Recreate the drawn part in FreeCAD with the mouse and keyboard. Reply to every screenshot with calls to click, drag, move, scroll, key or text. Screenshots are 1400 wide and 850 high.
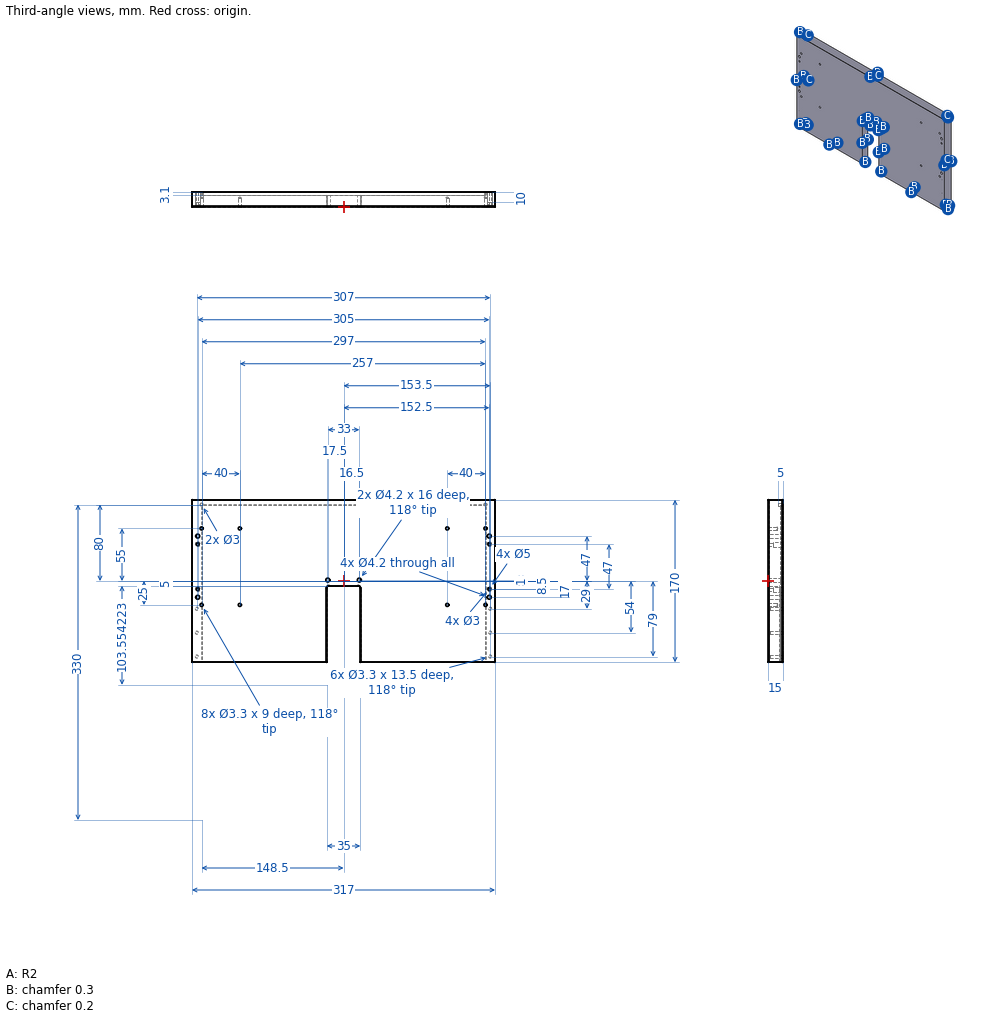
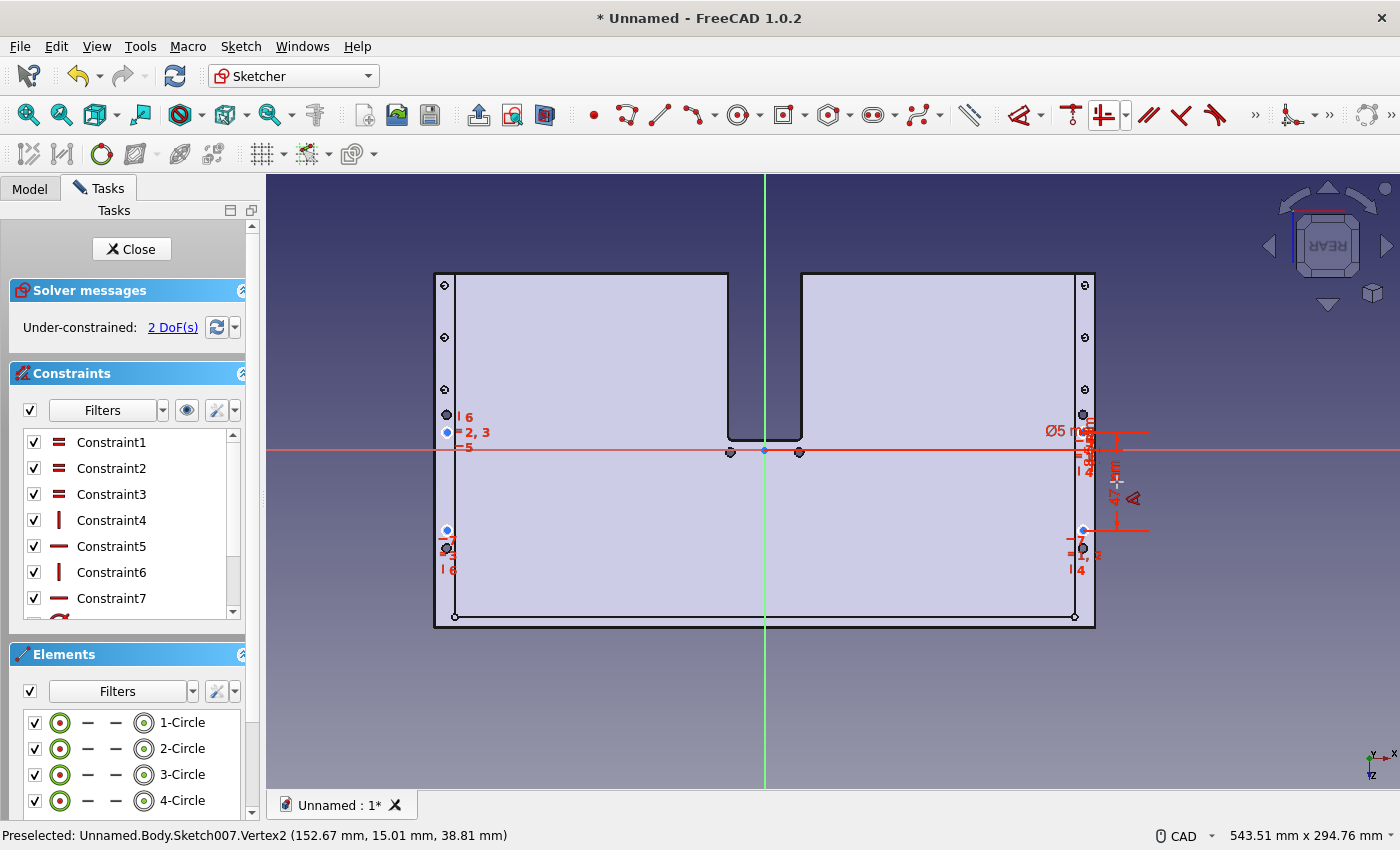
click(1083, 433)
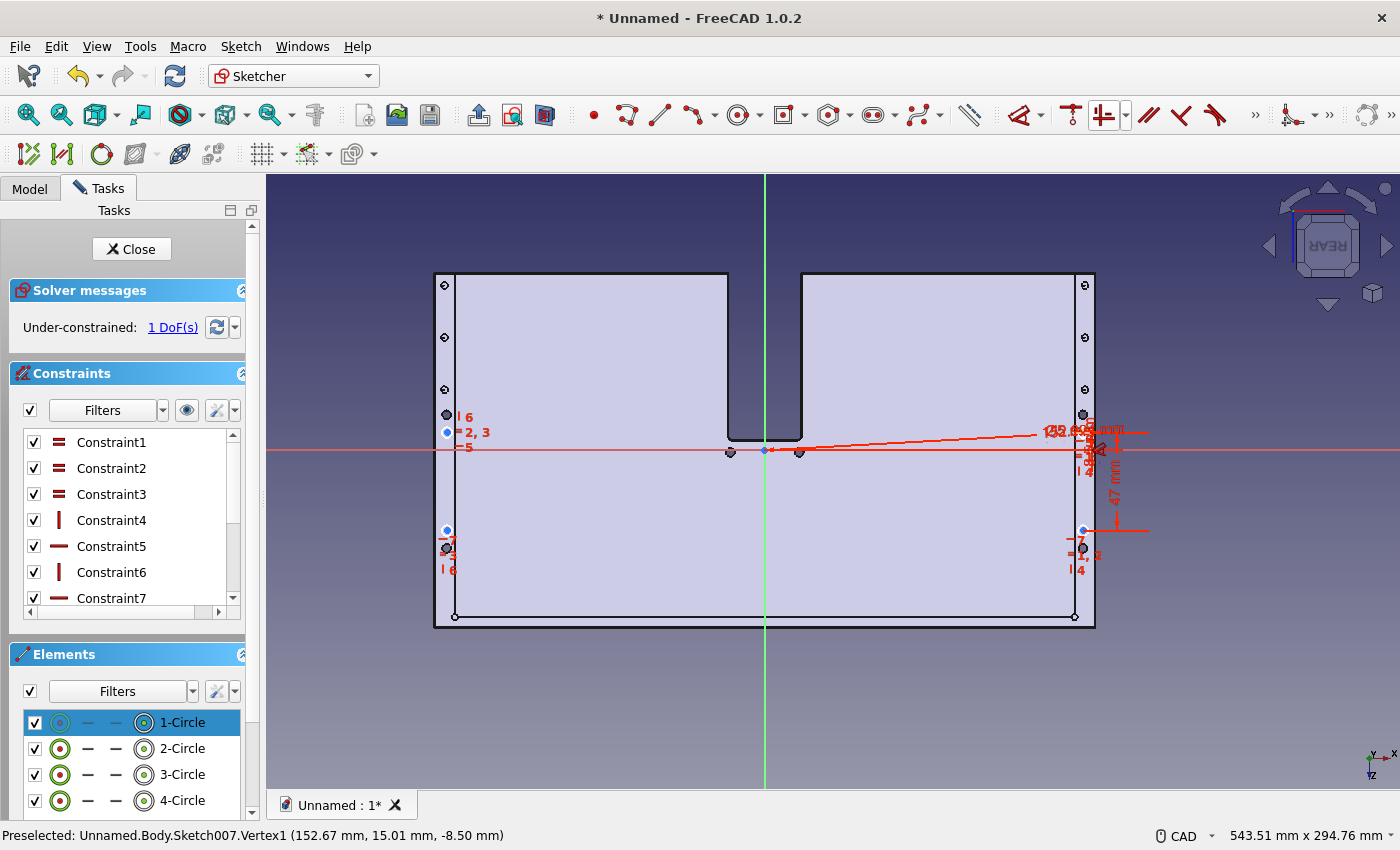
click(447, 433)
click(619, 399)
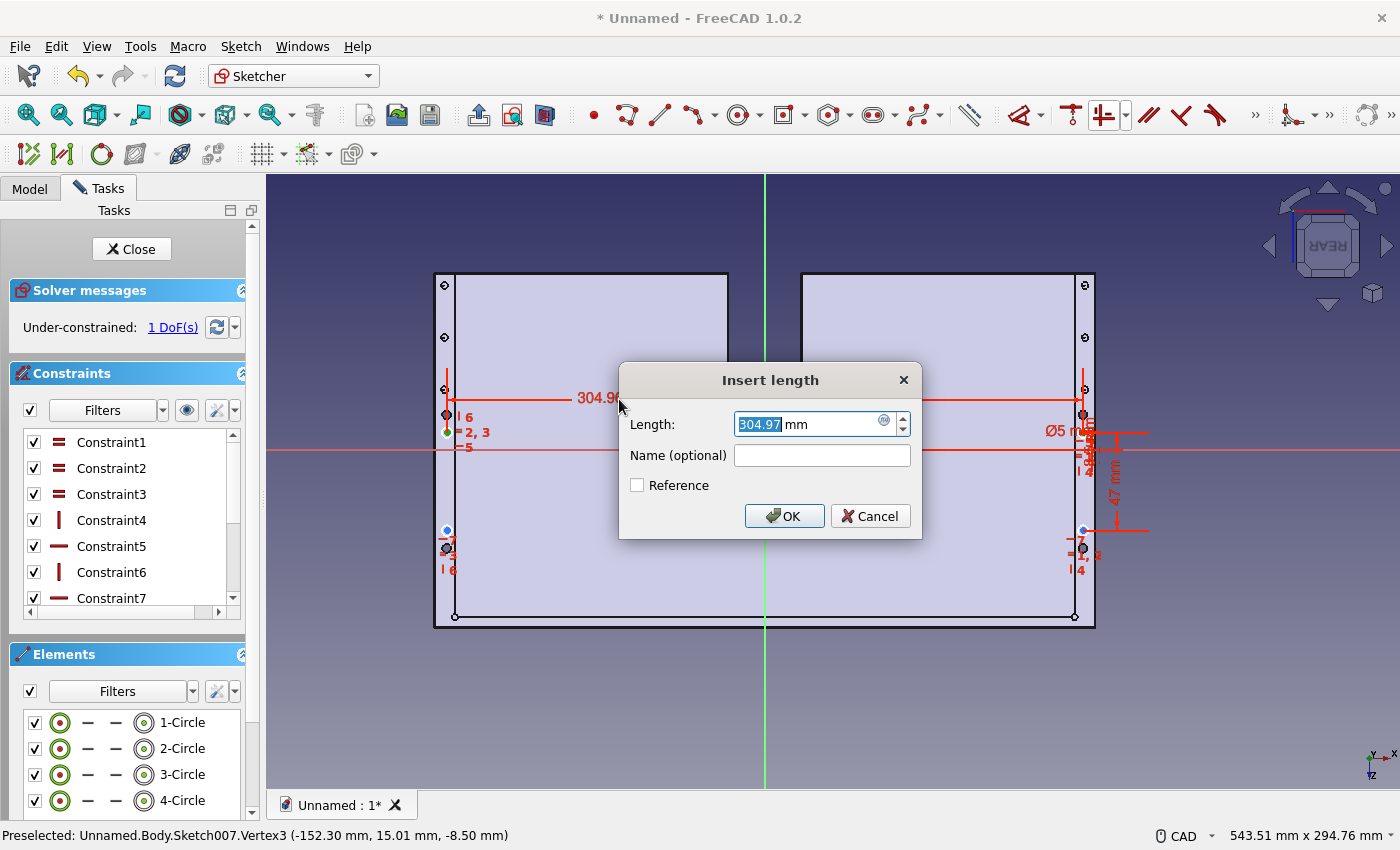
text(305)
key(Return)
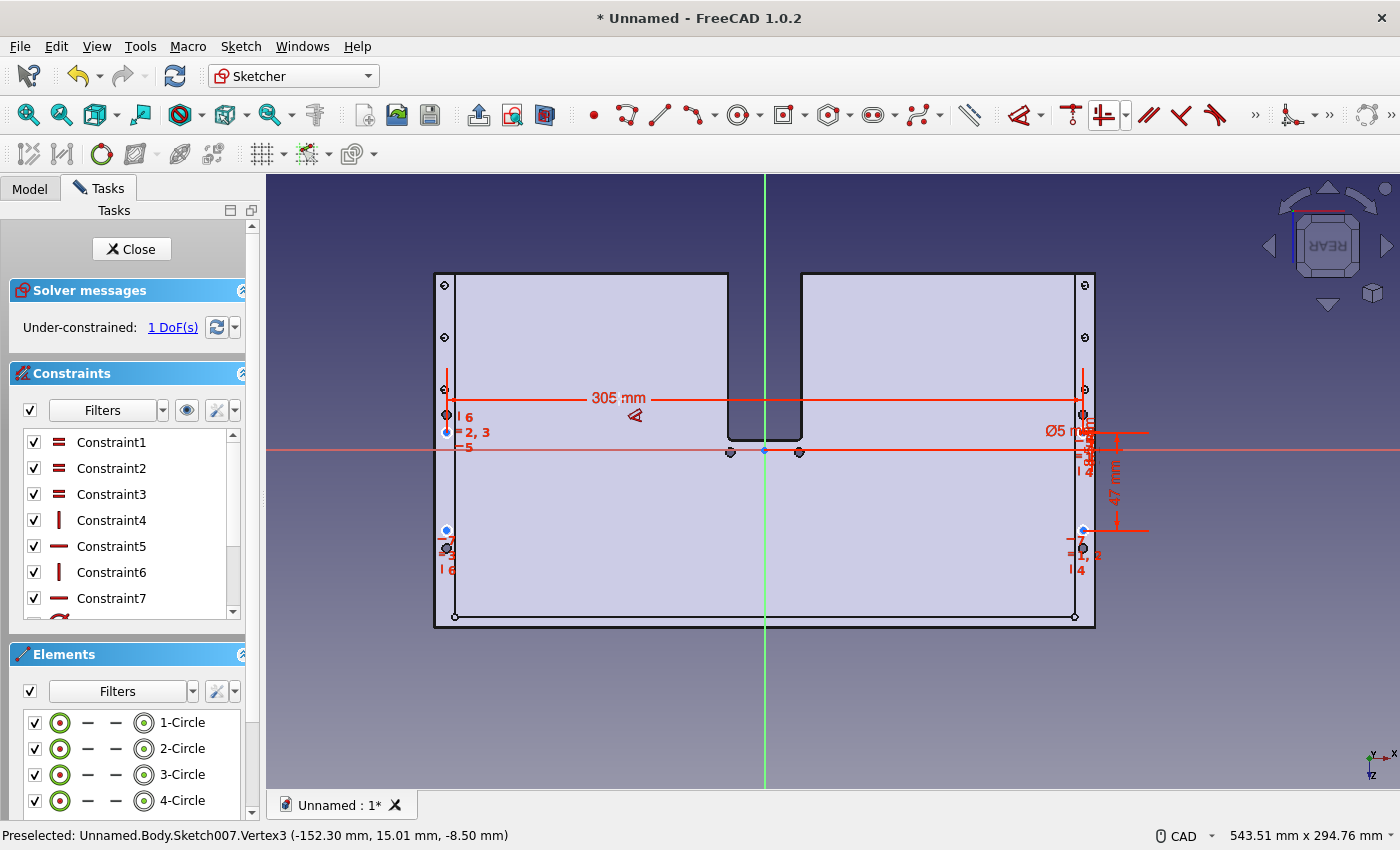
click(1083, 433)
click(924, 399)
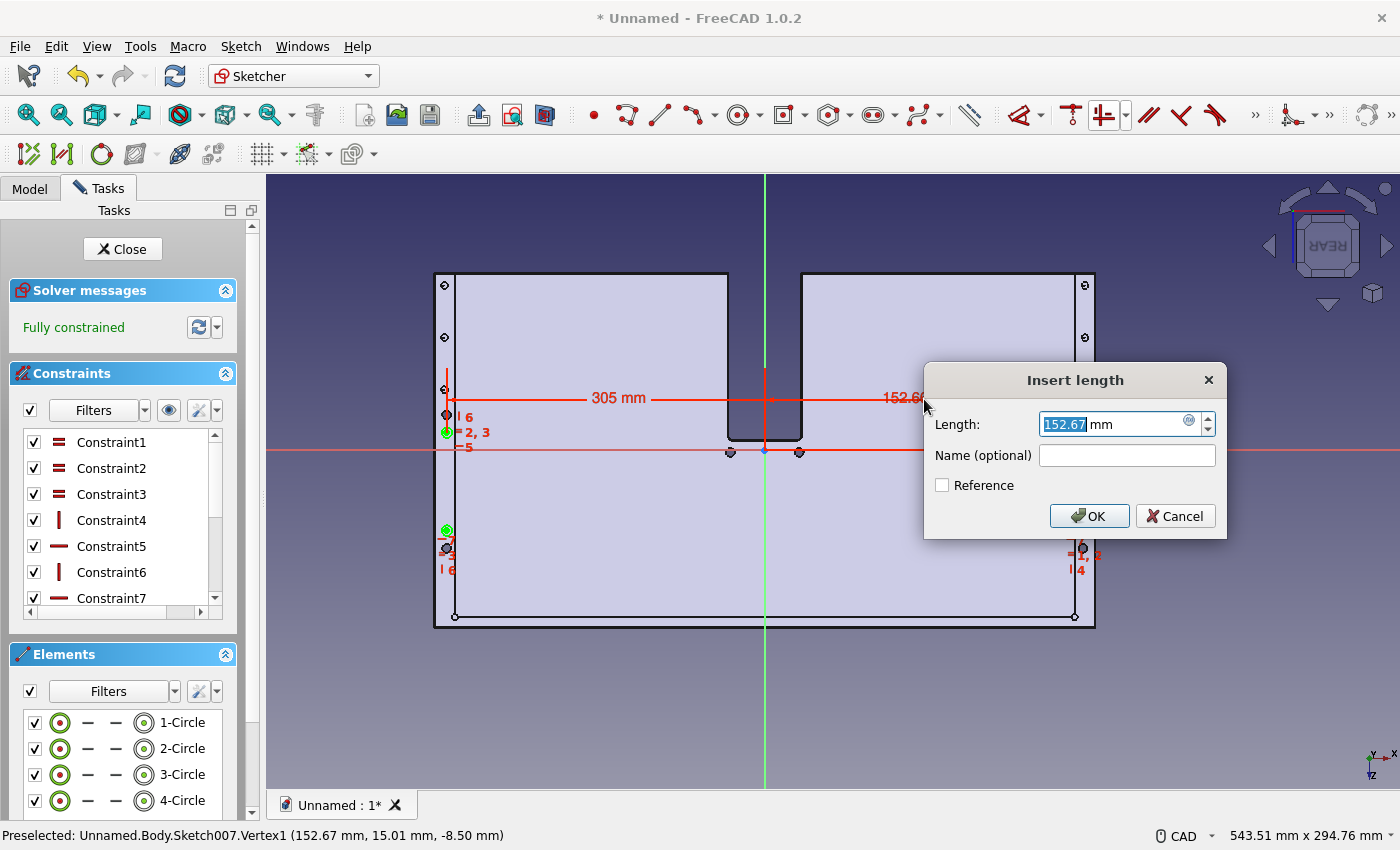
text(152.5)
key(Return)
key(Escape)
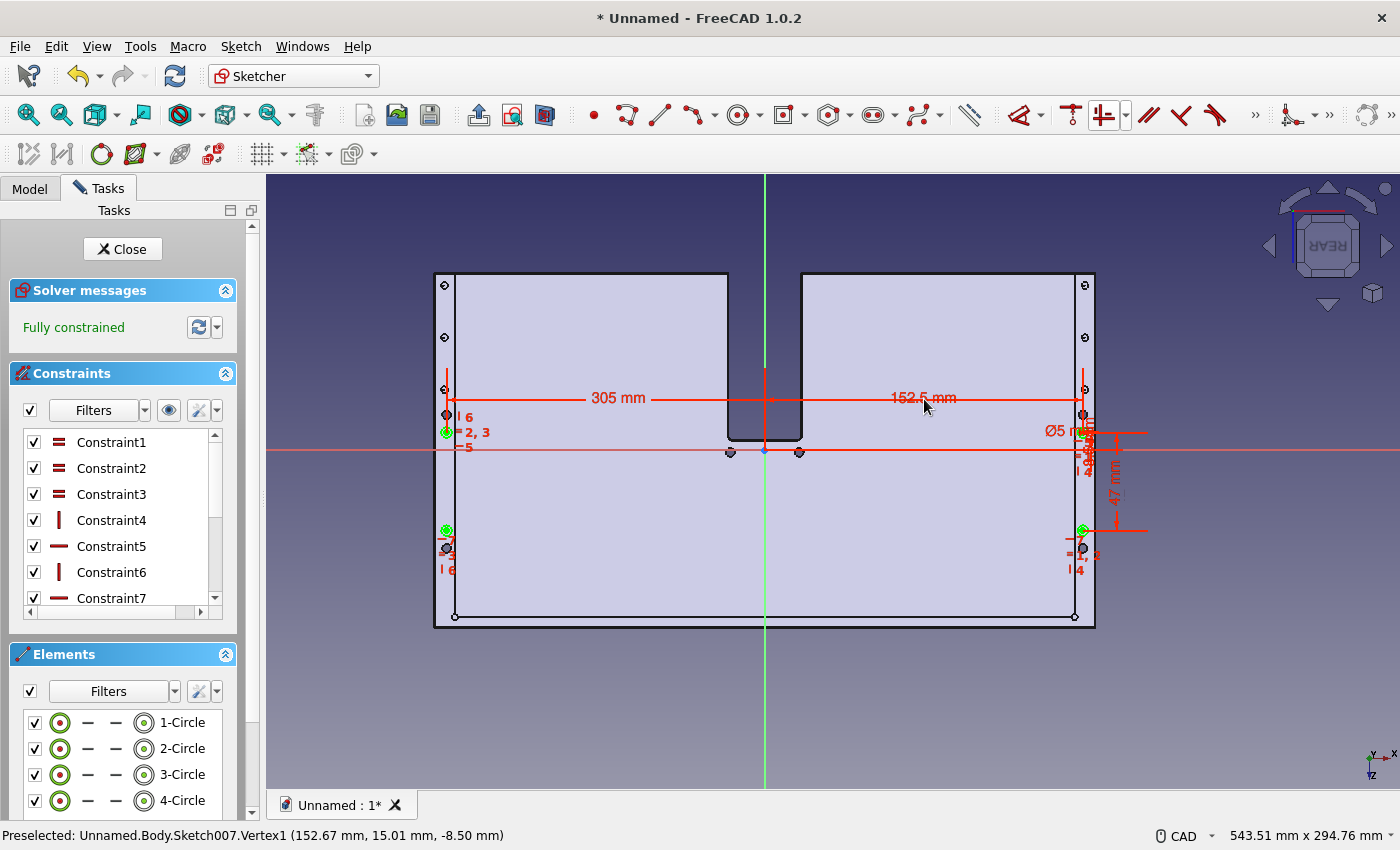
click(123, 249)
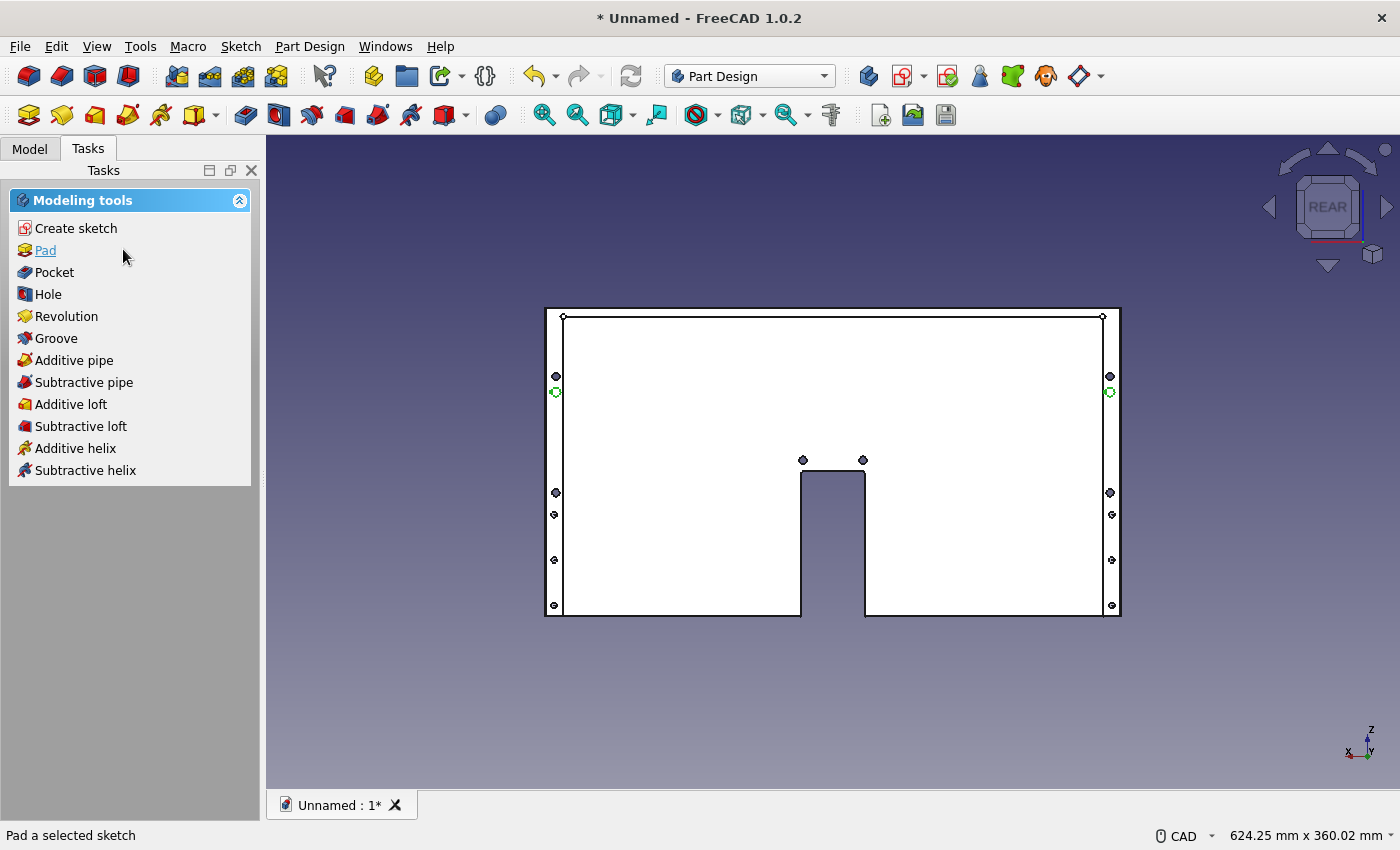
click(246, 116)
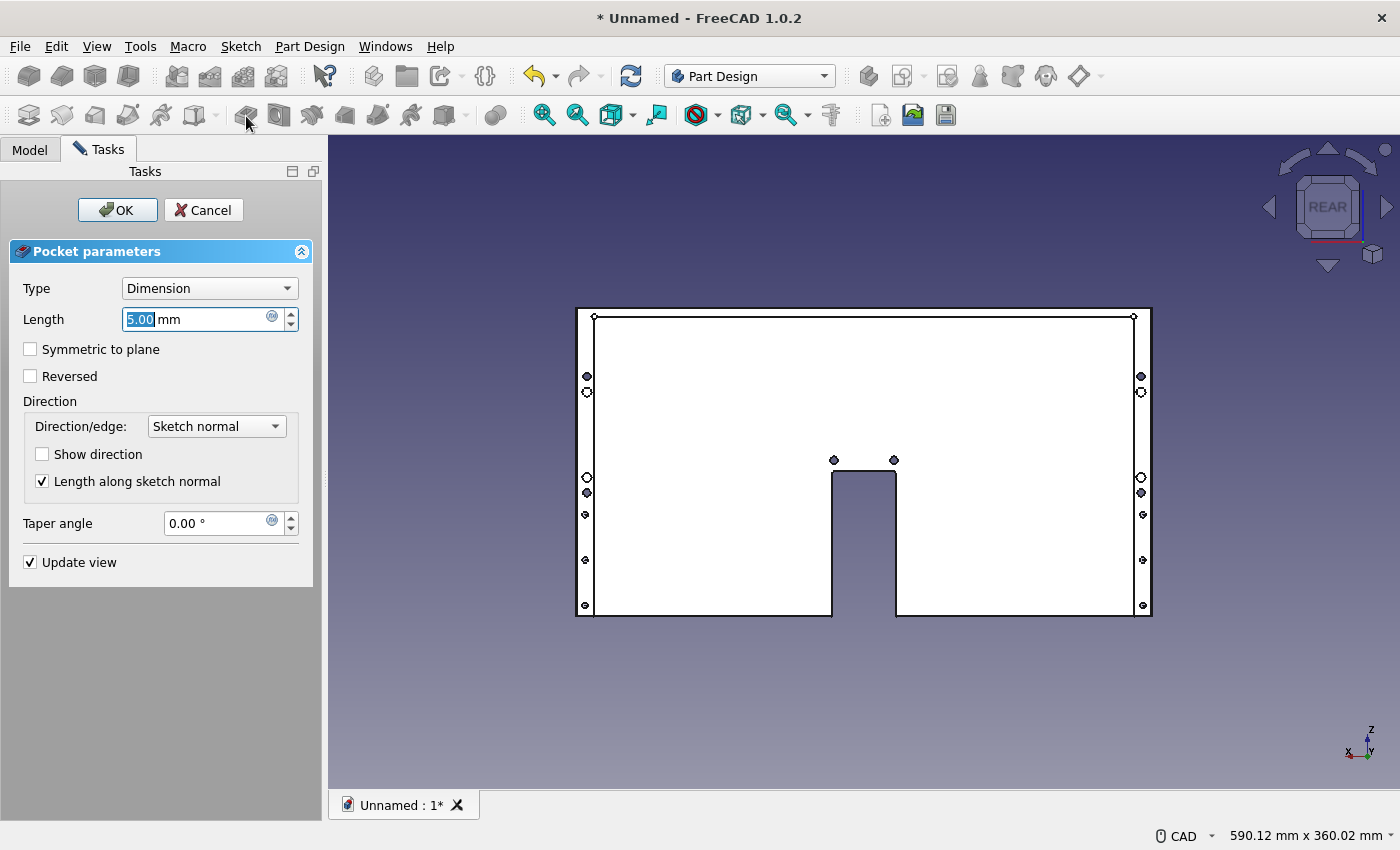
text(10)
key(Tab)